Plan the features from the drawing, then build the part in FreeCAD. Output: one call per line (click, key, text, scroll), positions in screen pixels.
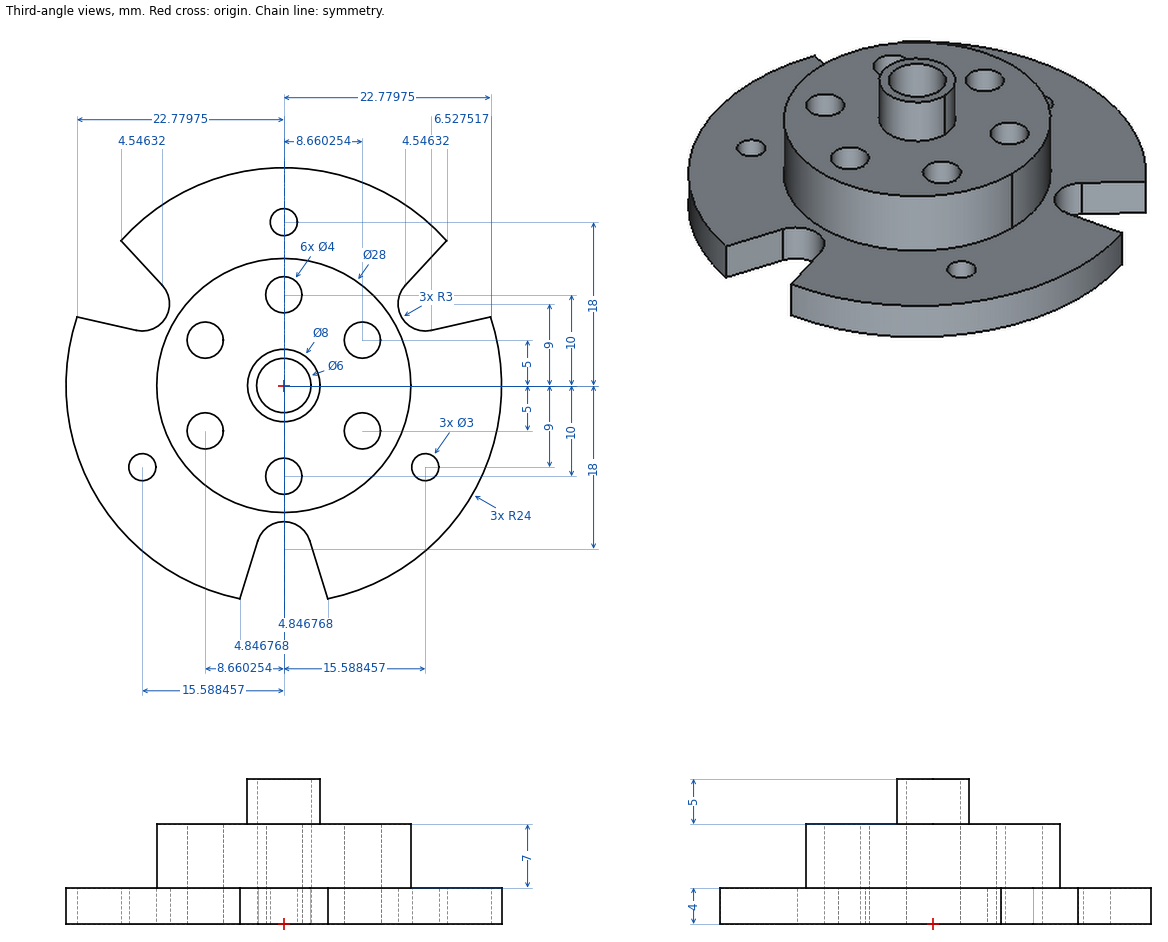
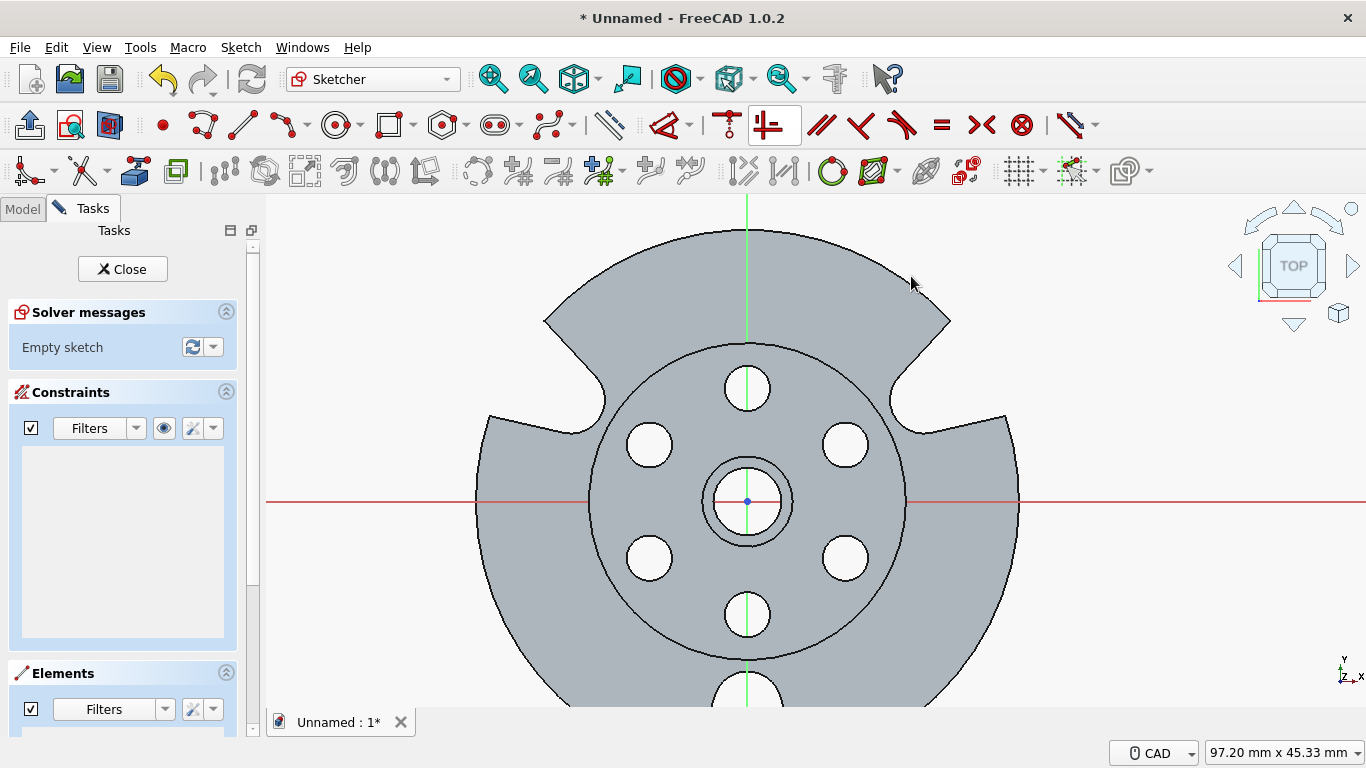
click(336, 126)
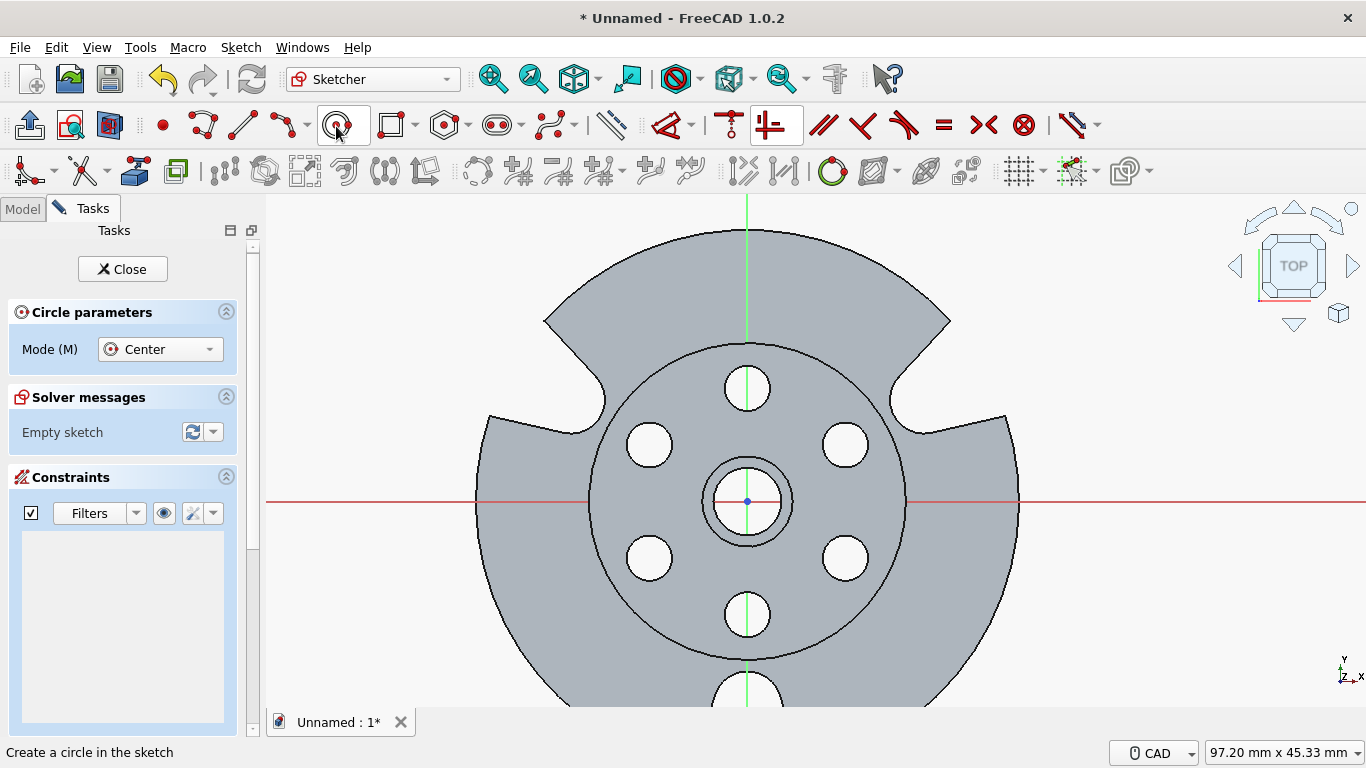
scroll(924, 603, up, 2)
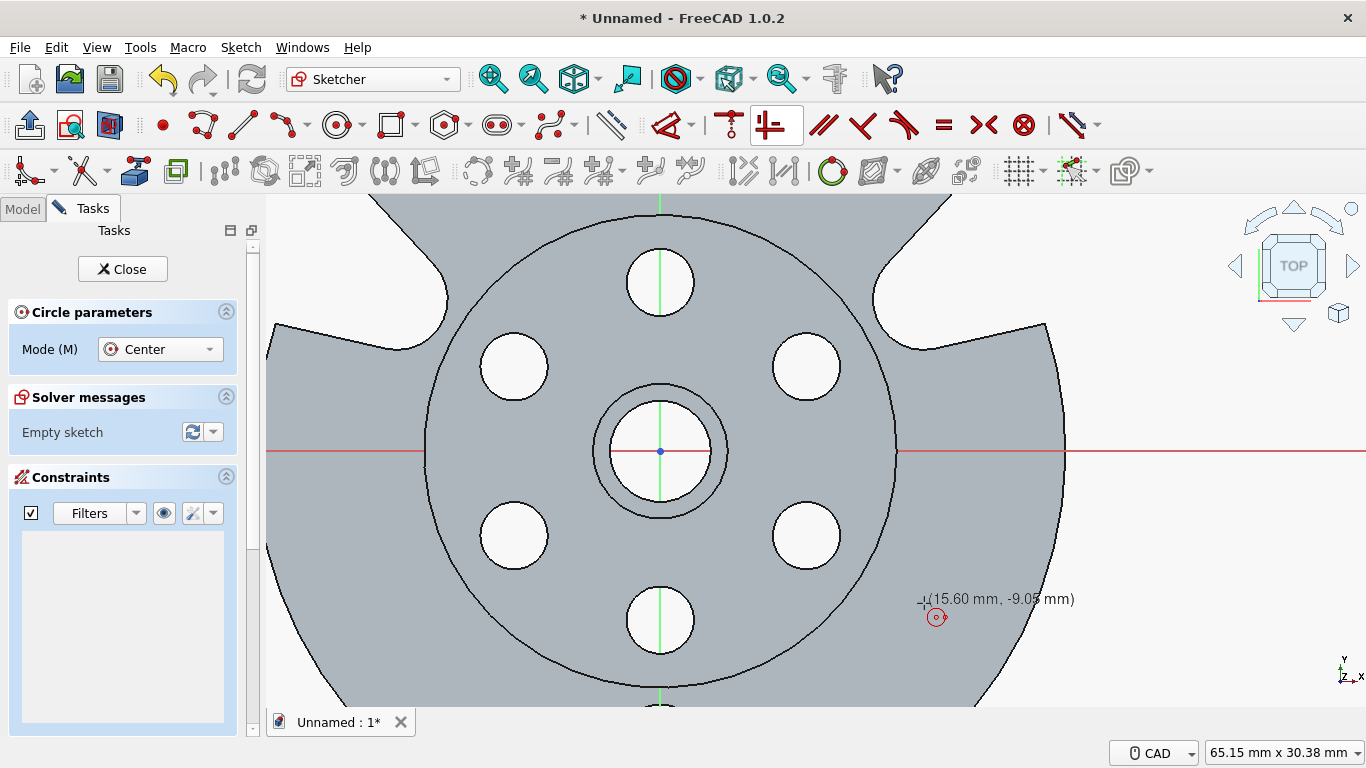
click(923, 603)
click(941, 585)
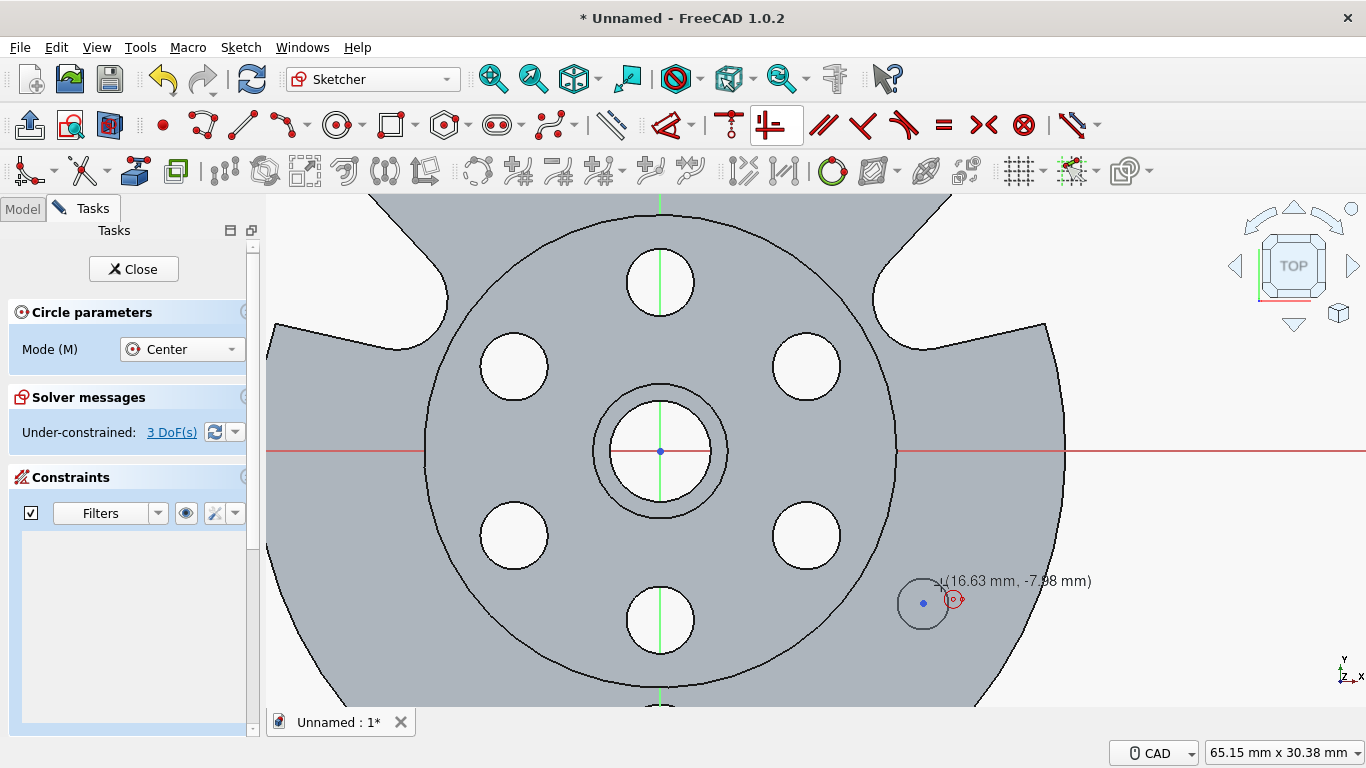
scroll(925, 603, down, 2)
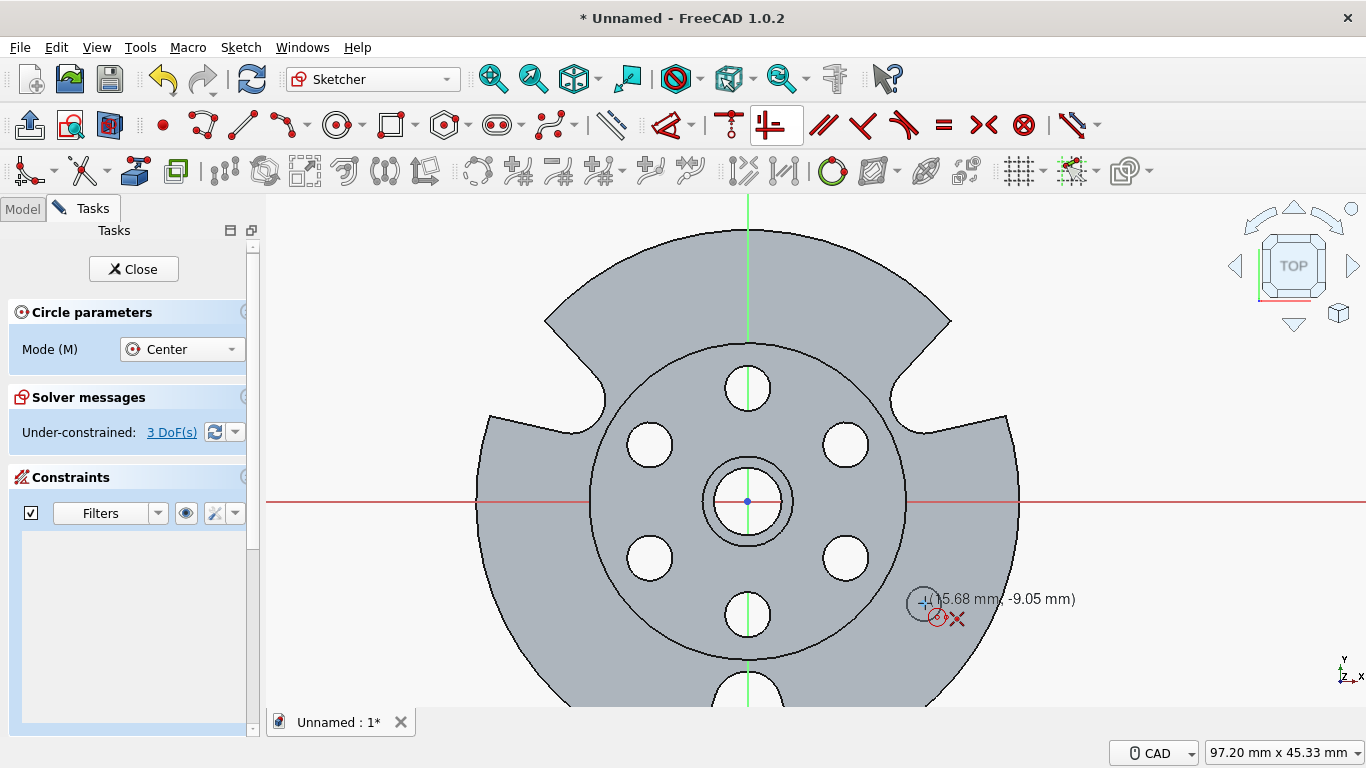
scroll(748, 298, up, 2)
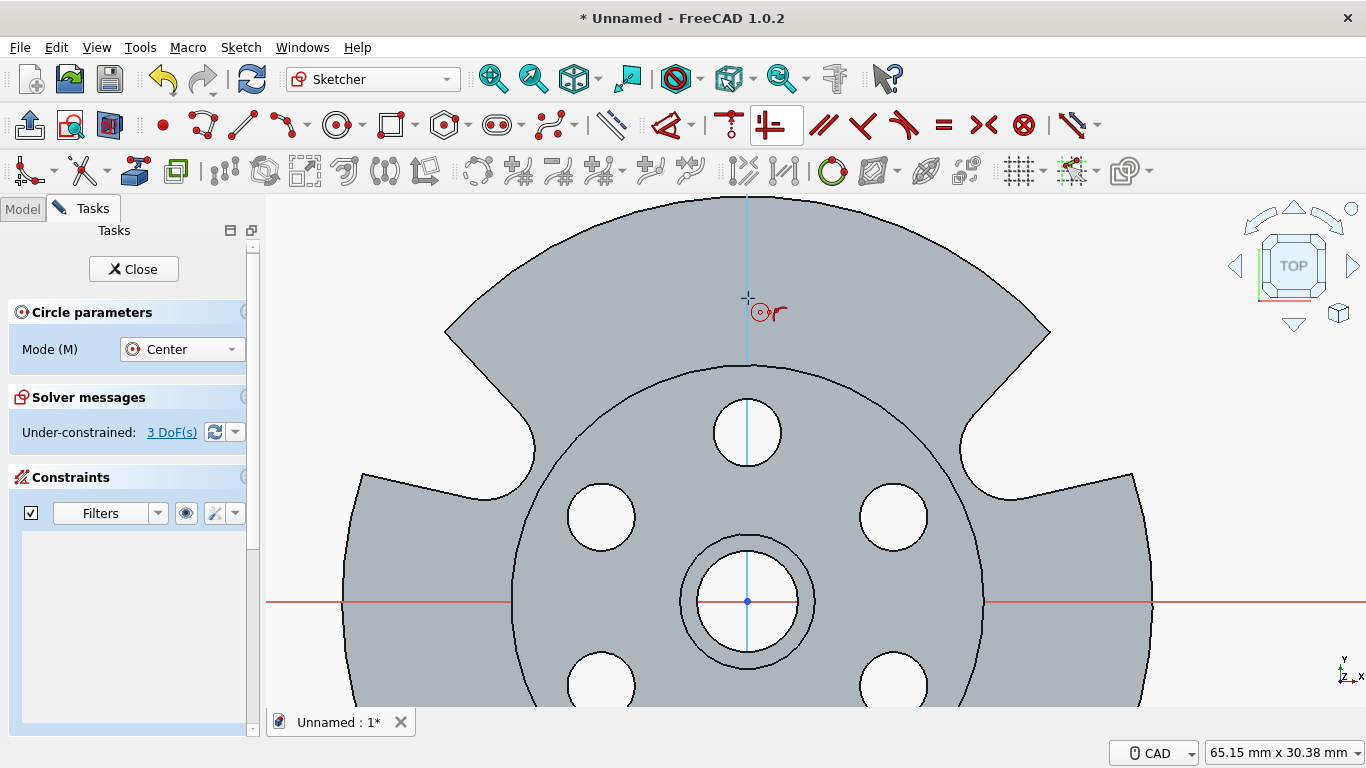
click(747, 298)
click(765, 280)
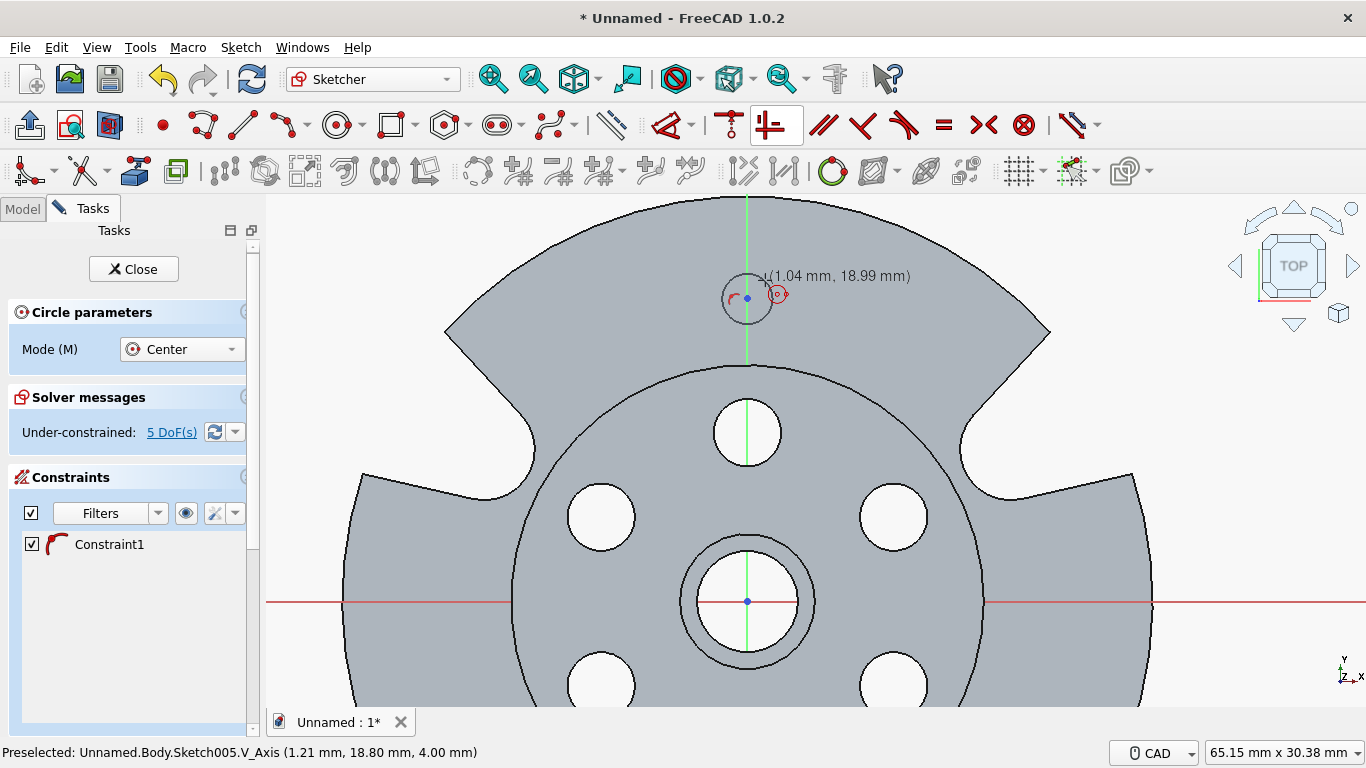
scroll(748, 298, down, 2)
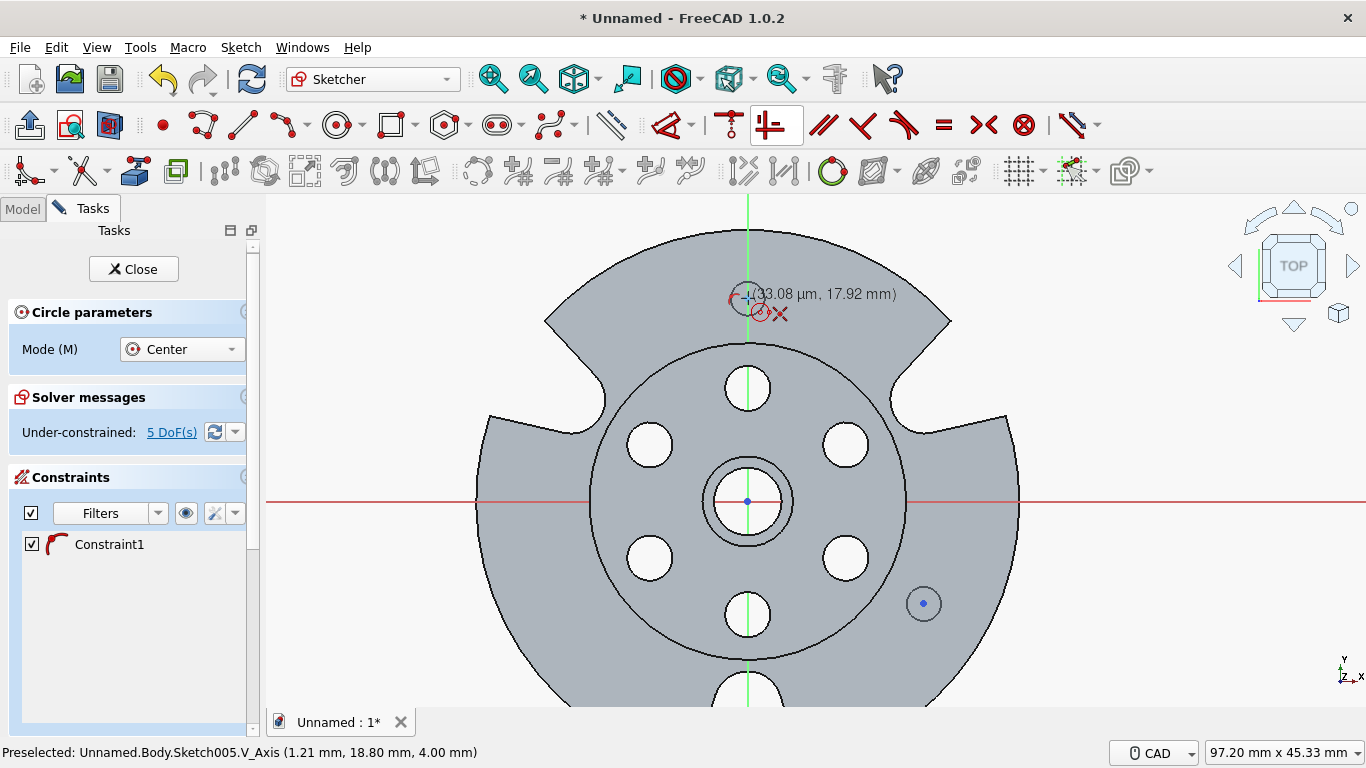
scroll(571, 603, up, 2)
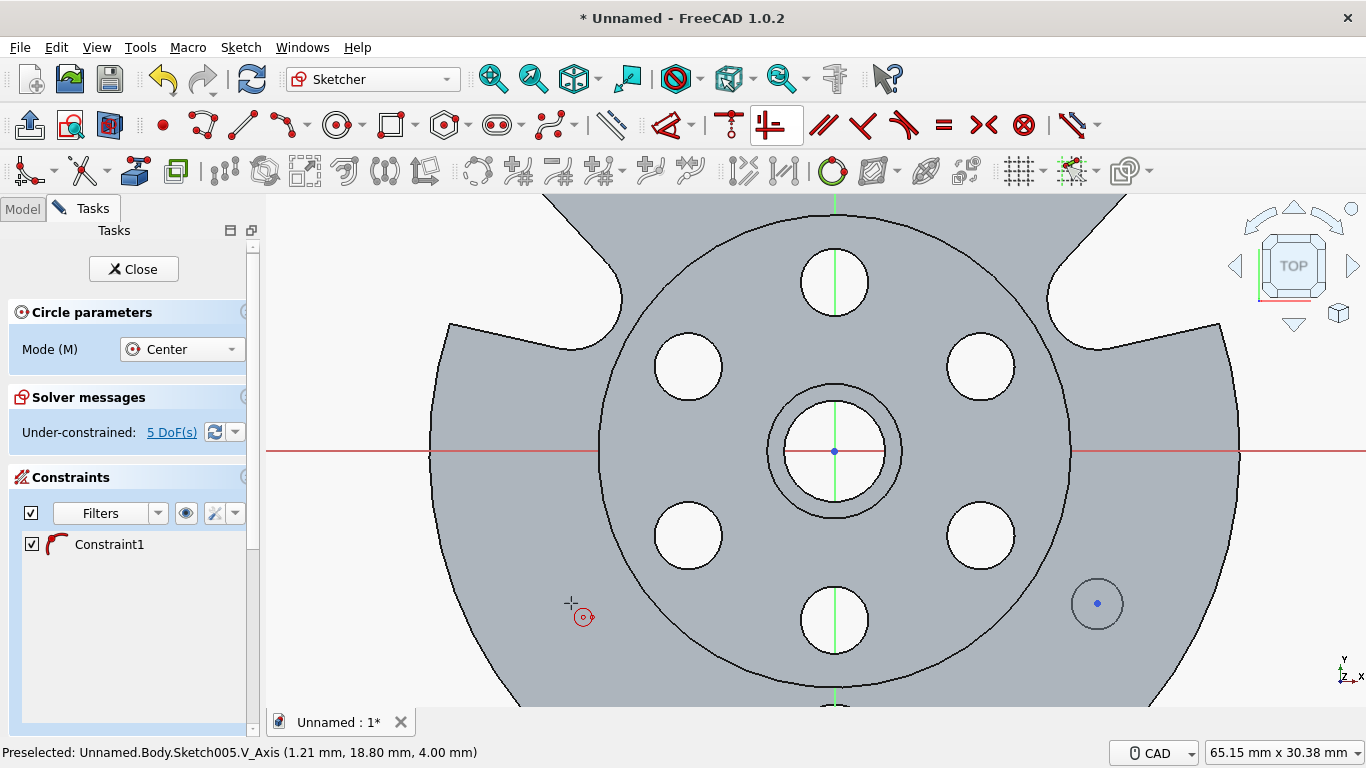
click(571, 603)
click(589, 585)
key(Escape)